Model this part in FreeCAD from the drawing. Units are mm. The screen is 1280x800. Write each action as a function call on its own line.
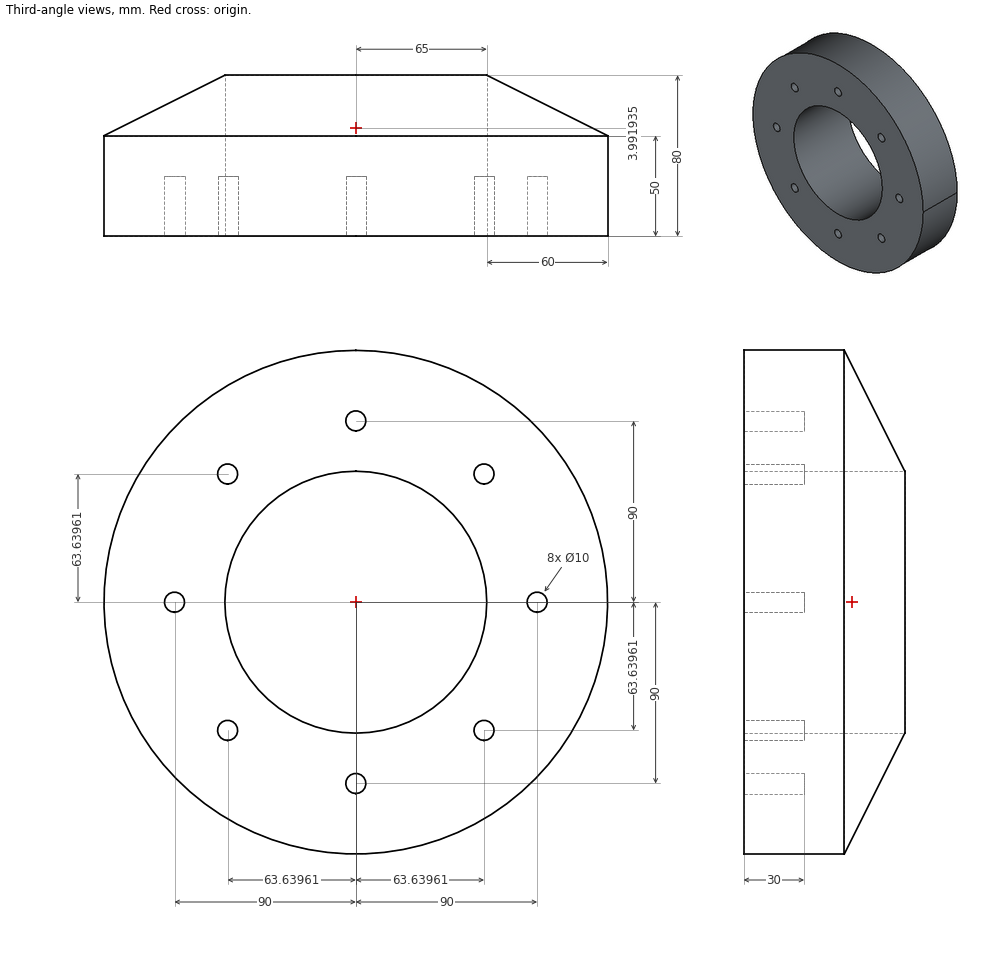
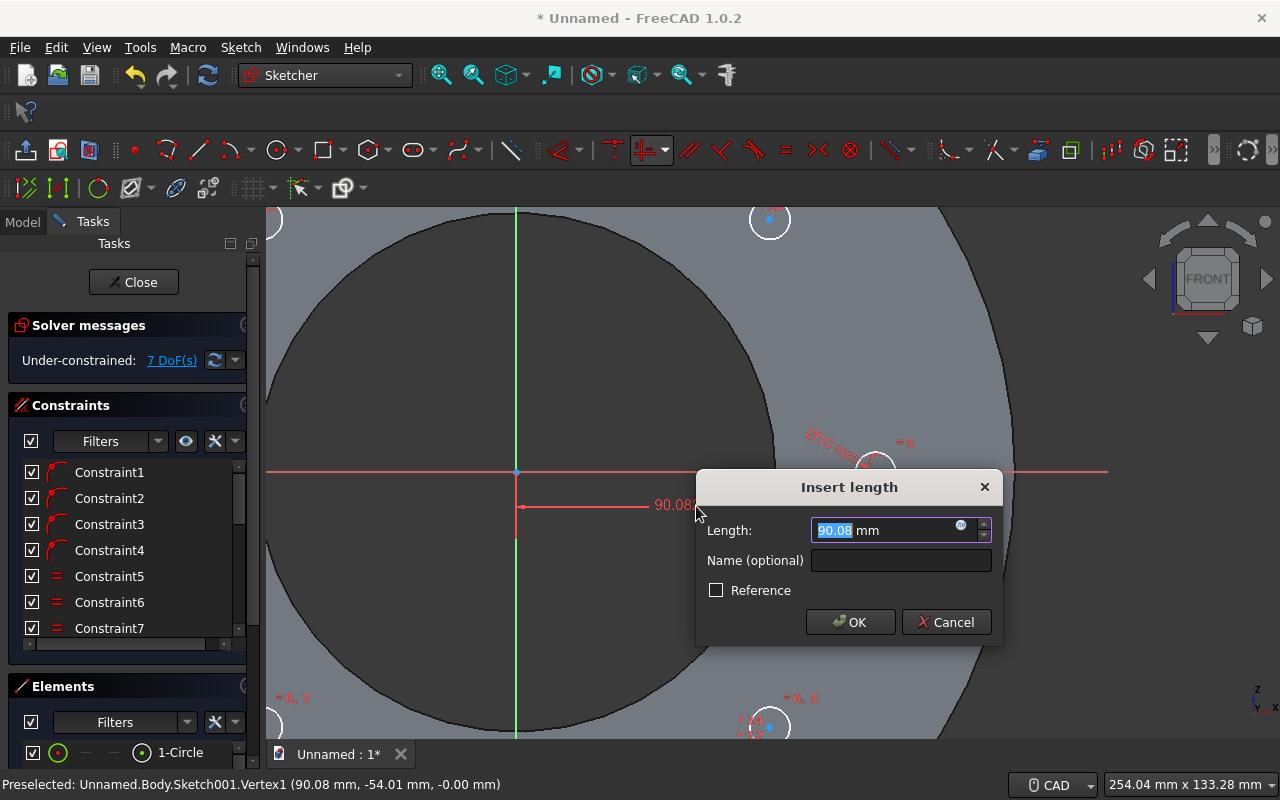
text(90)
key(Return)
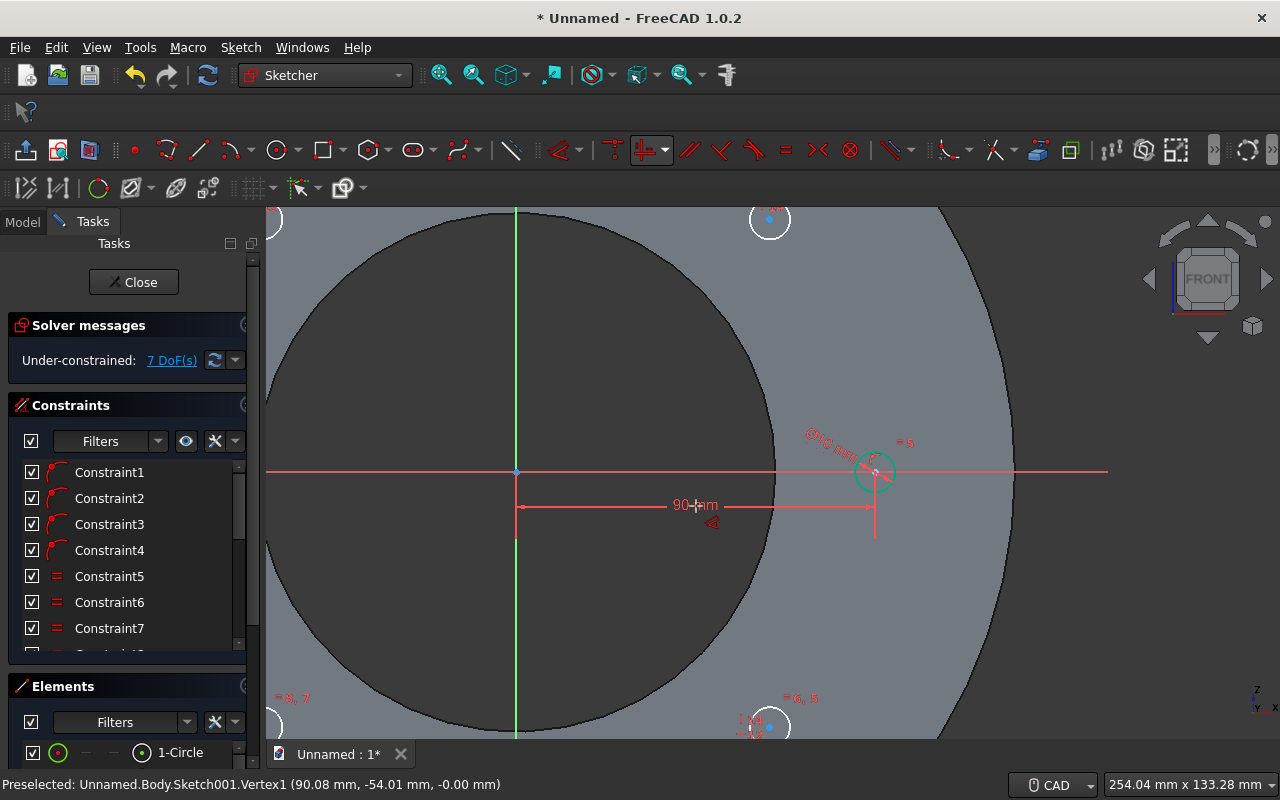
scroll(858, 474, down, 4)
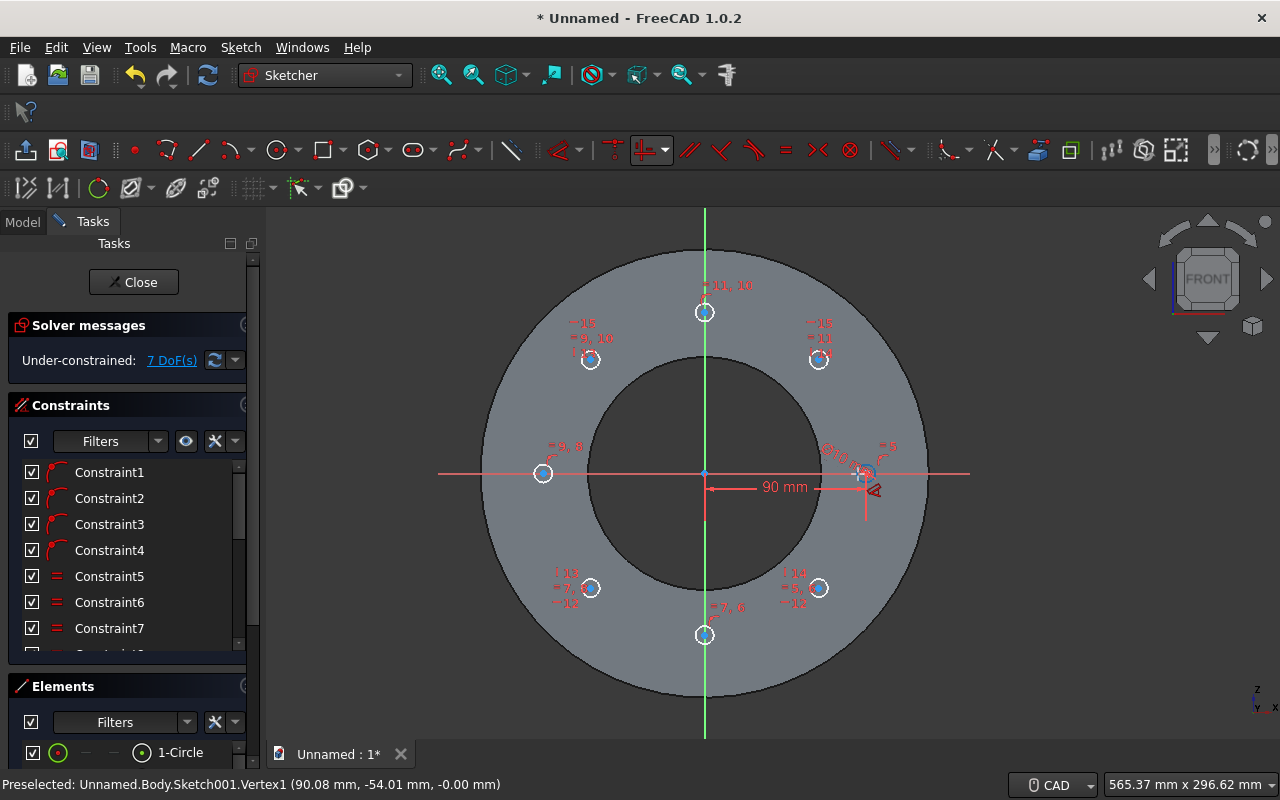
click(705, 635)
click(739, 554)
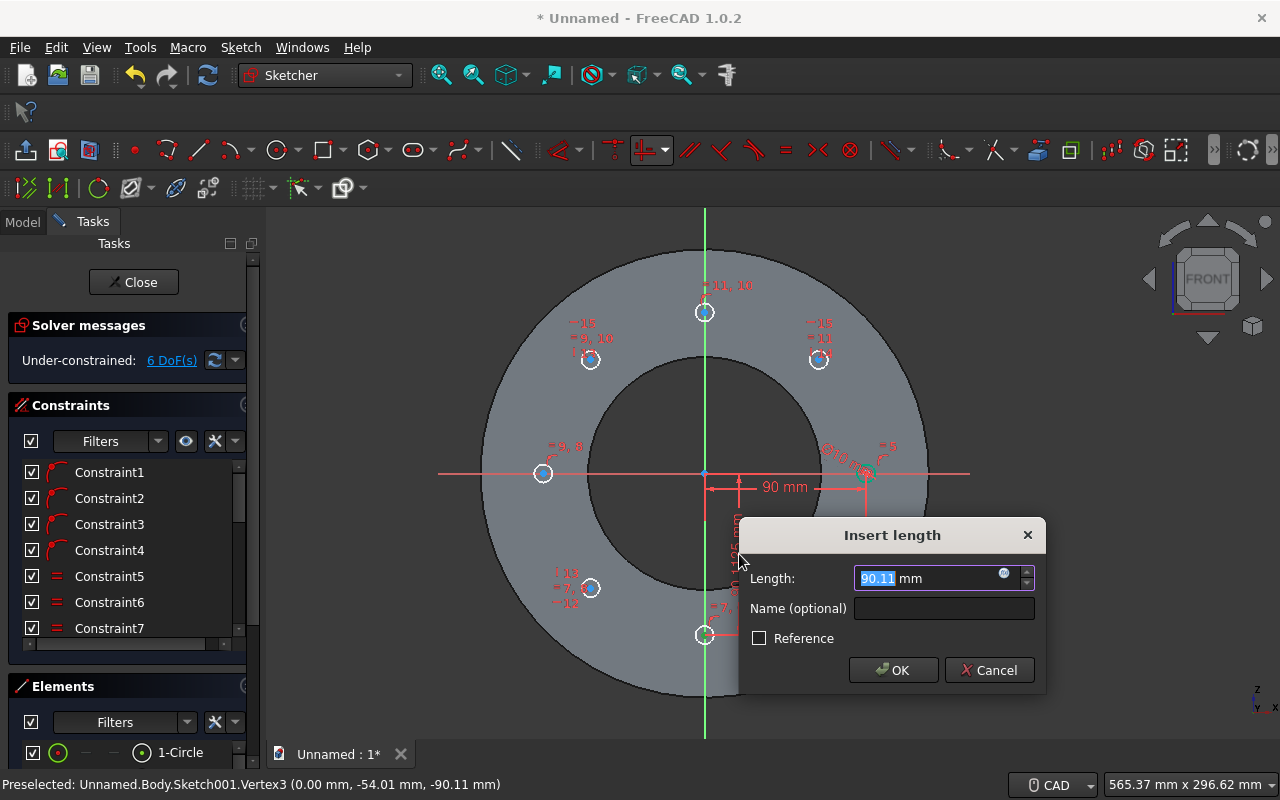
text(90)
key(Return)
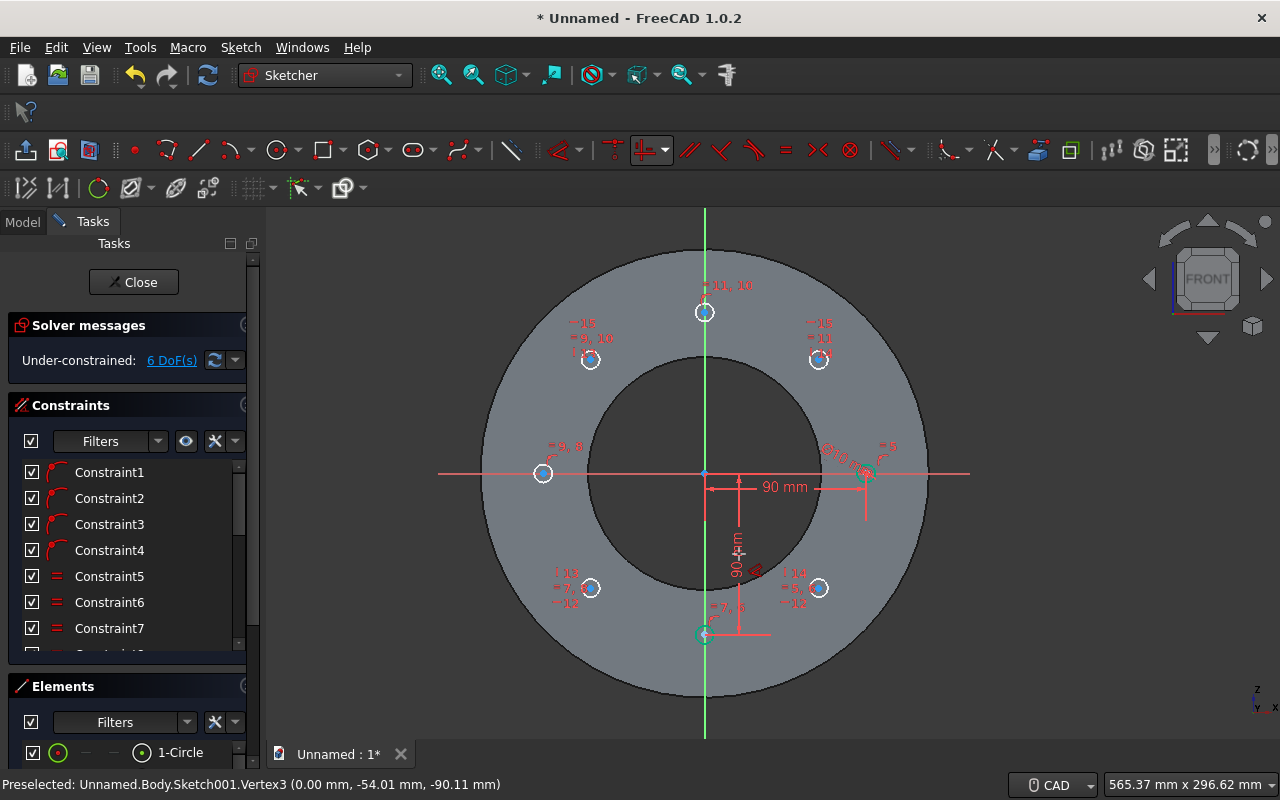
click(543, 474)
click(624, 508)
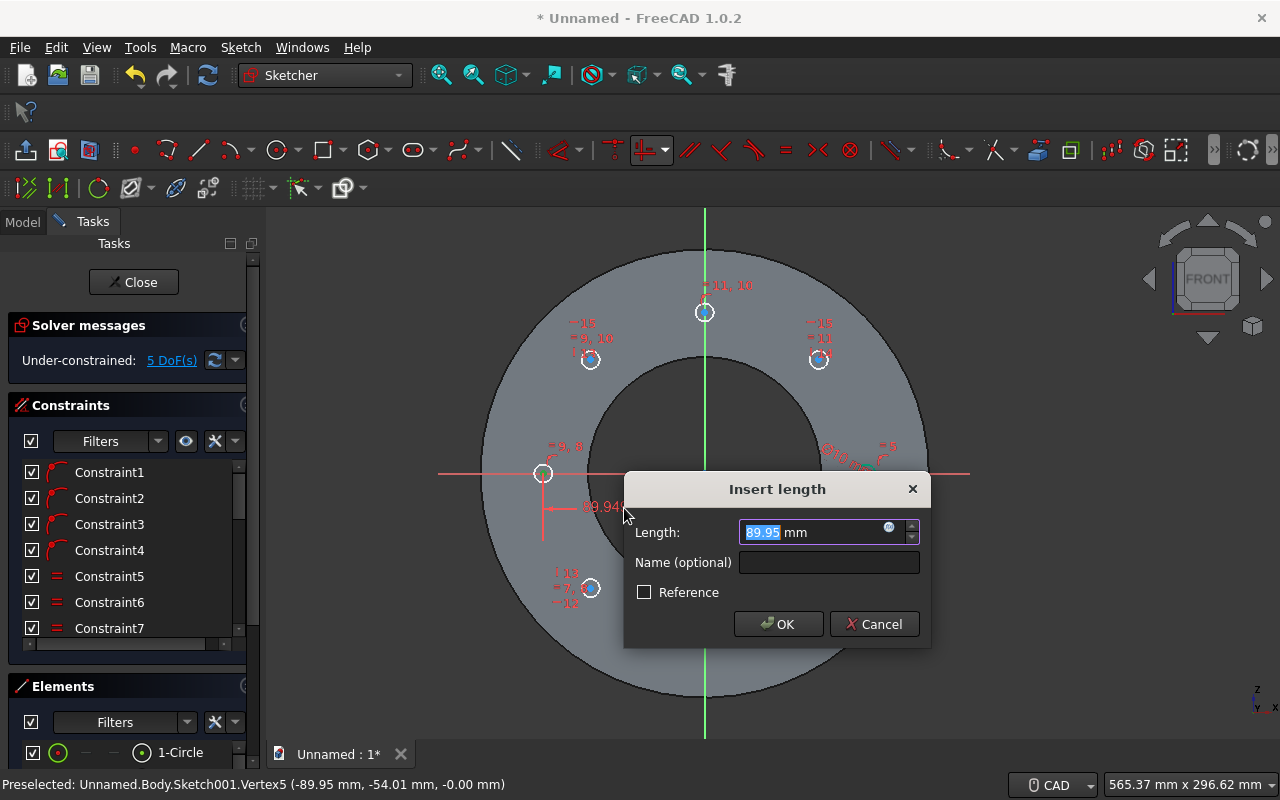
text(90)
key(Return)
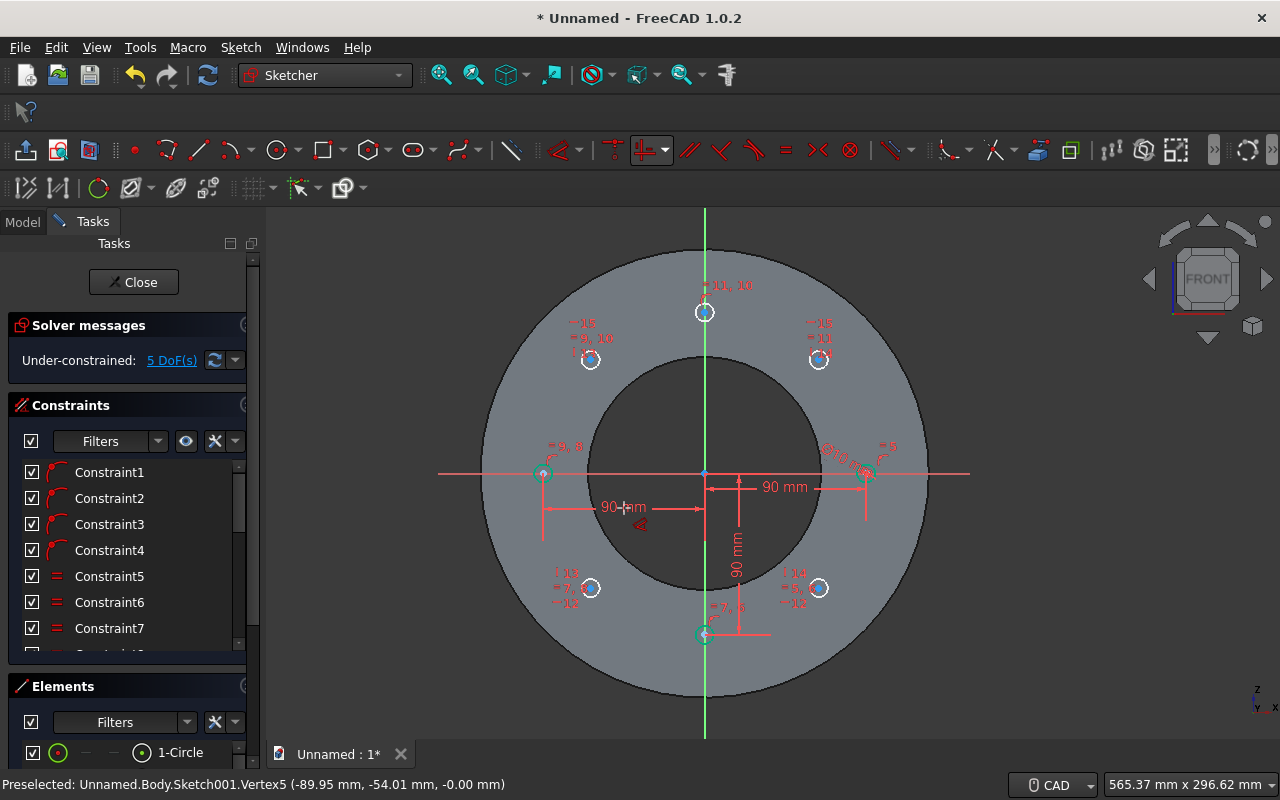
click(705, 312)
click(739, 393)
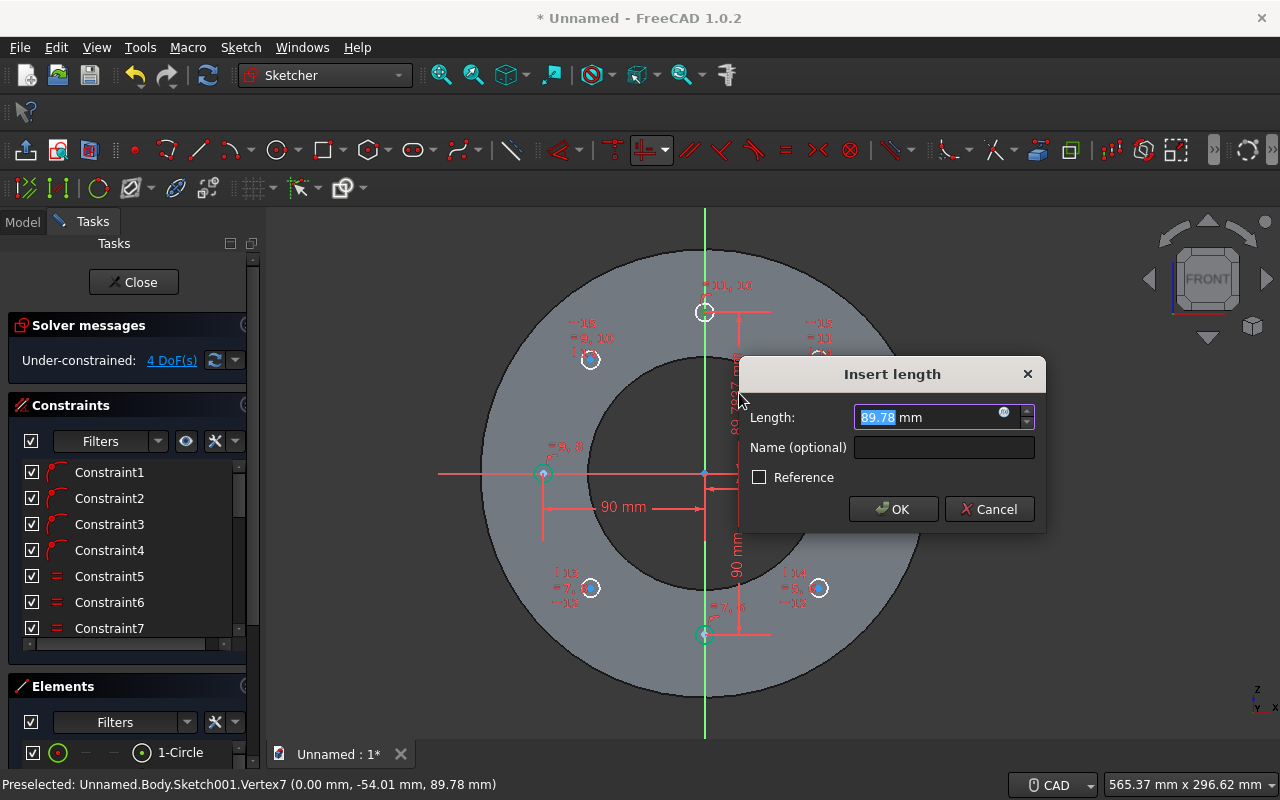
text(90)
key(Return)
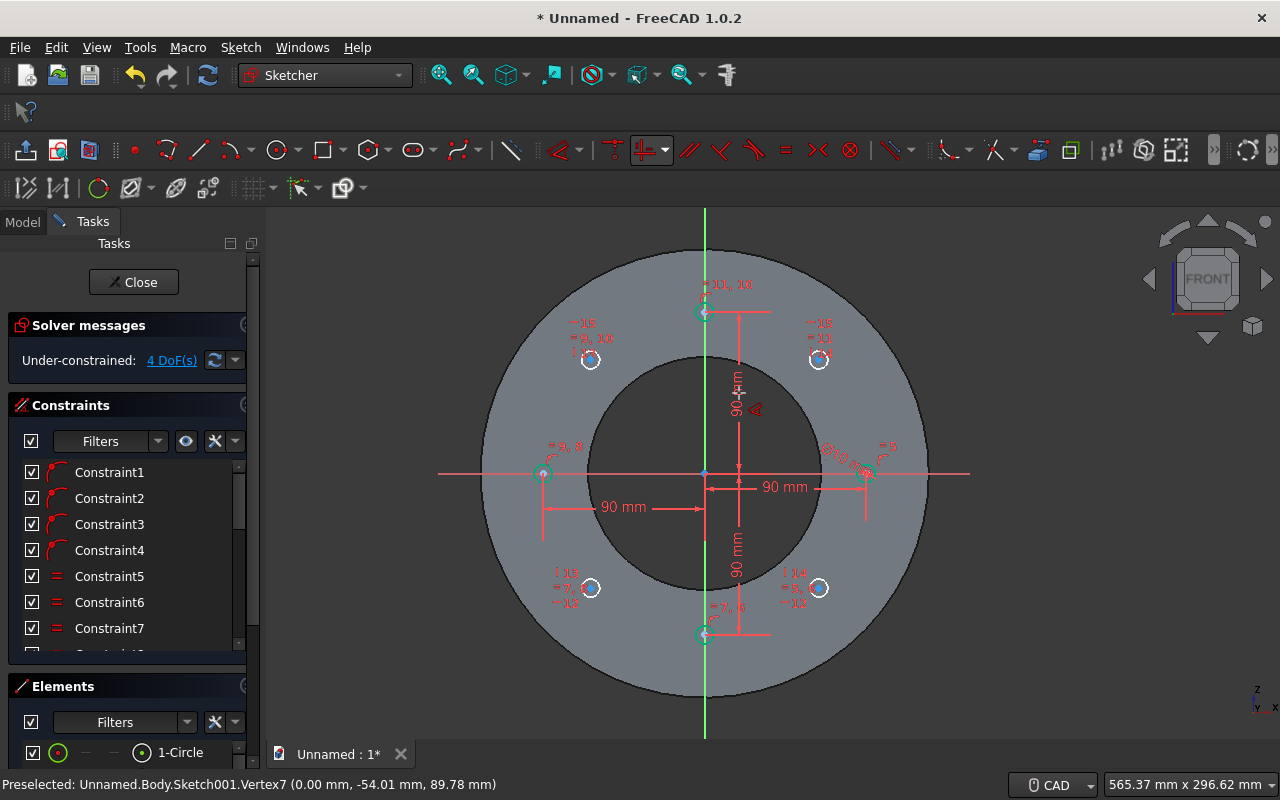
click(819, 588)
click(762, 622)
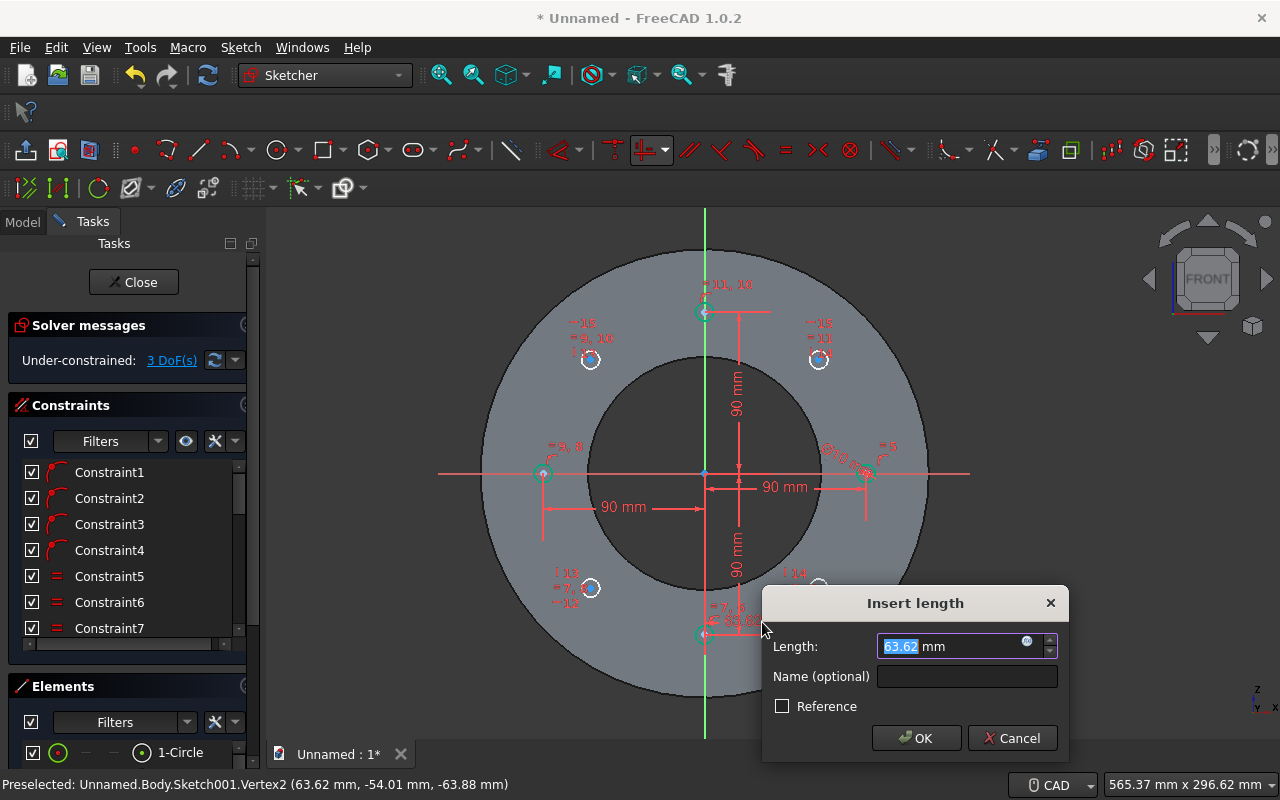
text(63.63961)
key(Return)